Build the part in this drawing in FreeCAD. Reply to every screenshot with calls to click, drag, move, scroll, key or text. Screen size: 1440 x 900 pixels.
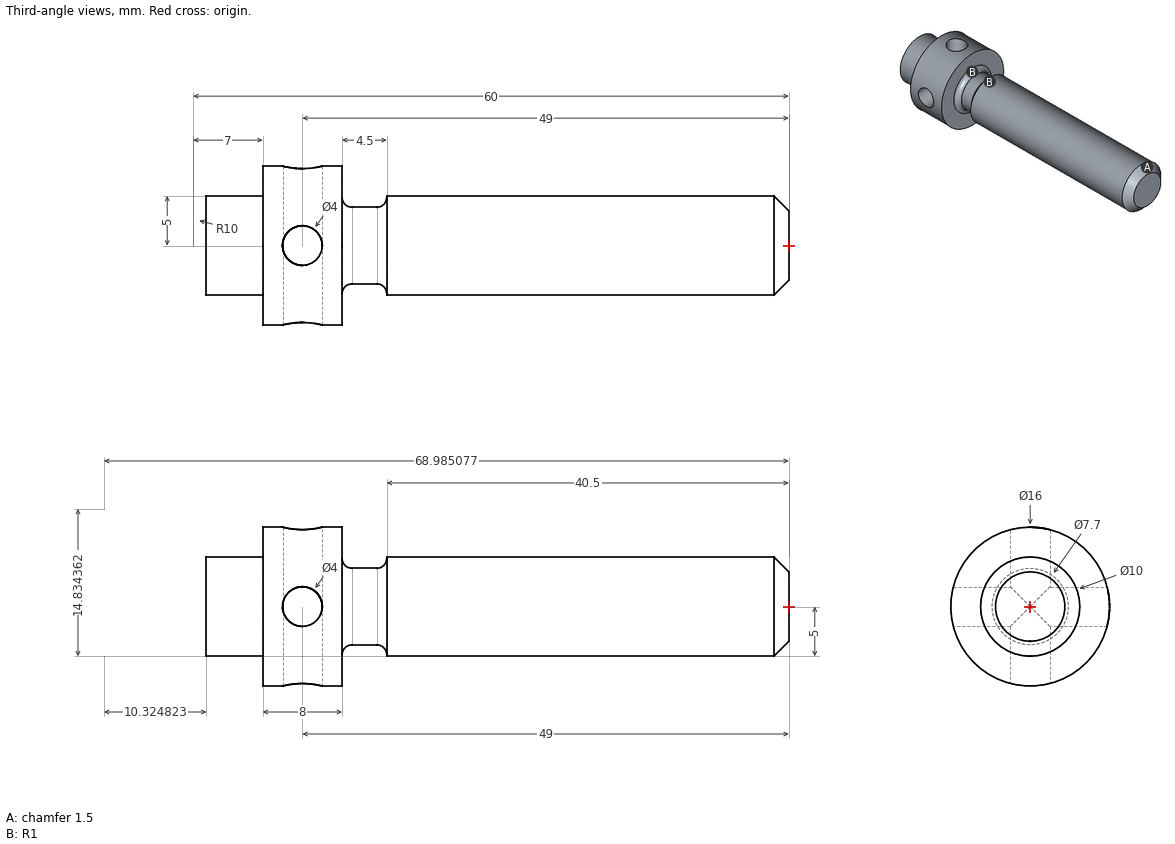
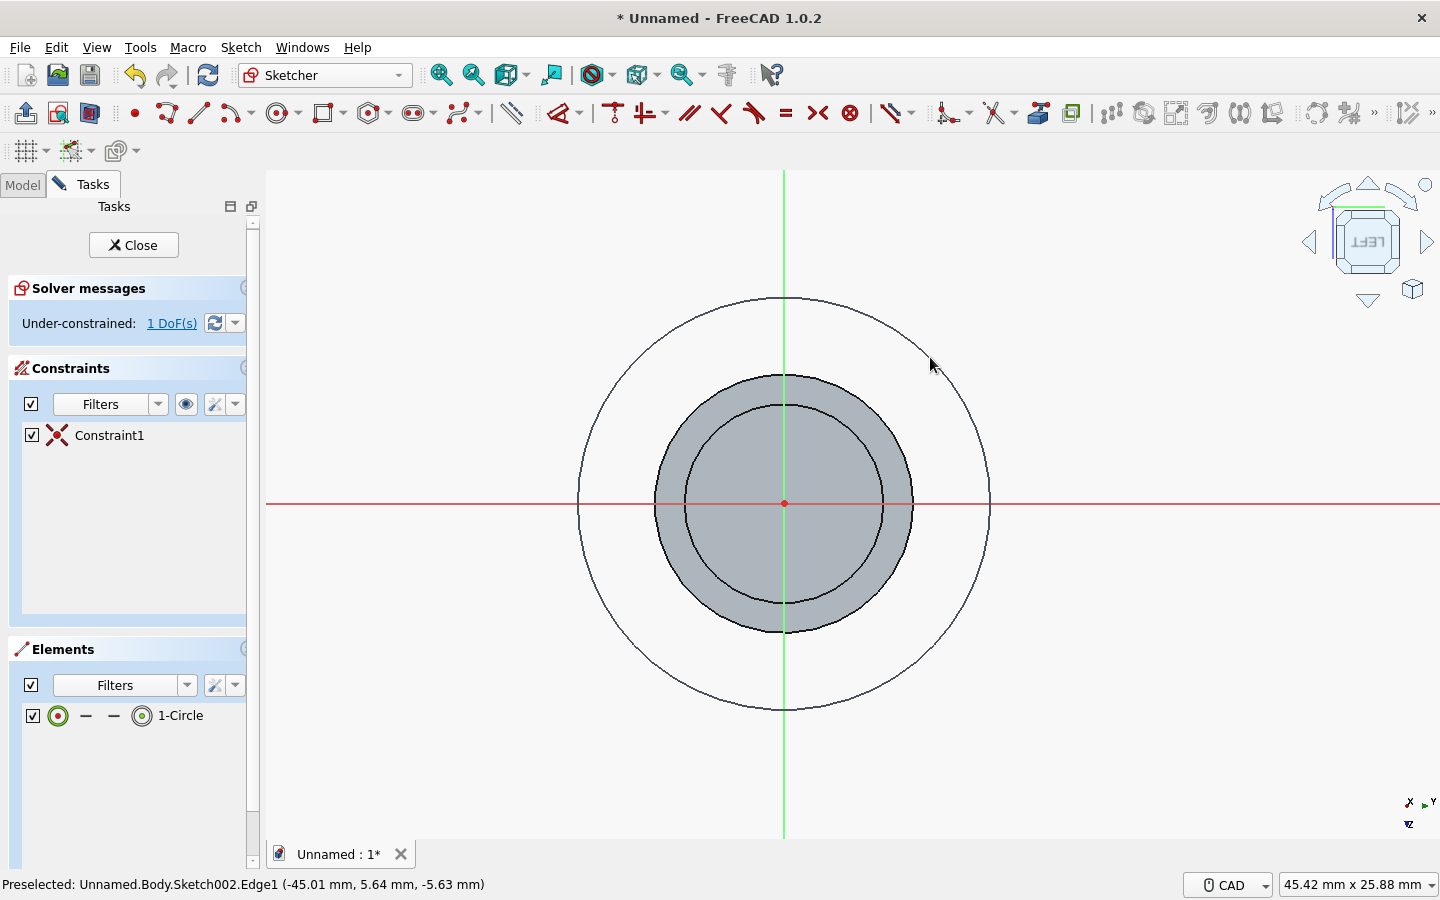
click(558, 114)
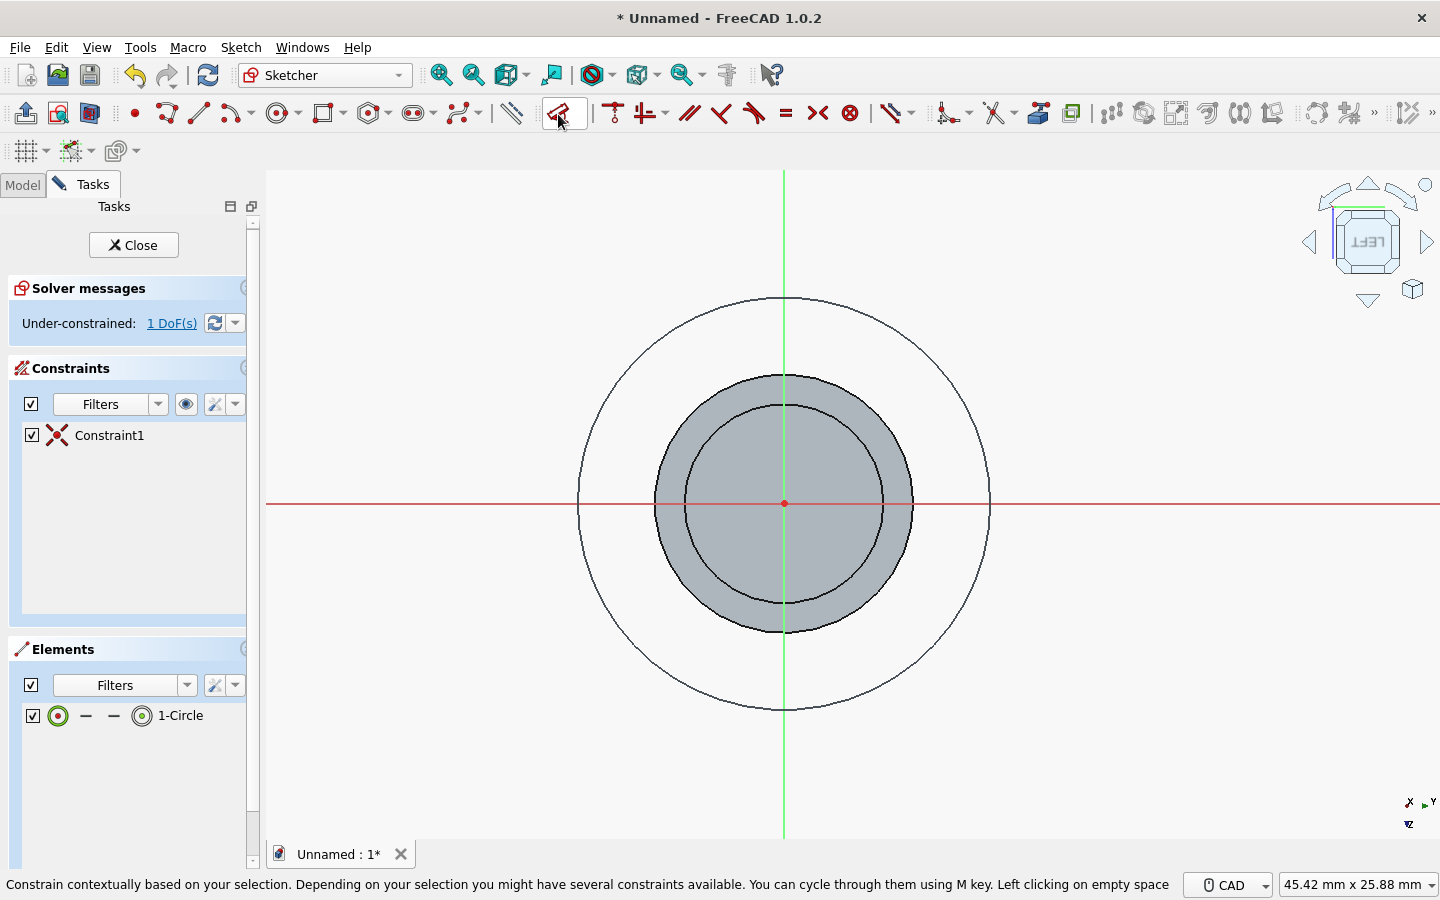
click(929, 357)
click(951, 334)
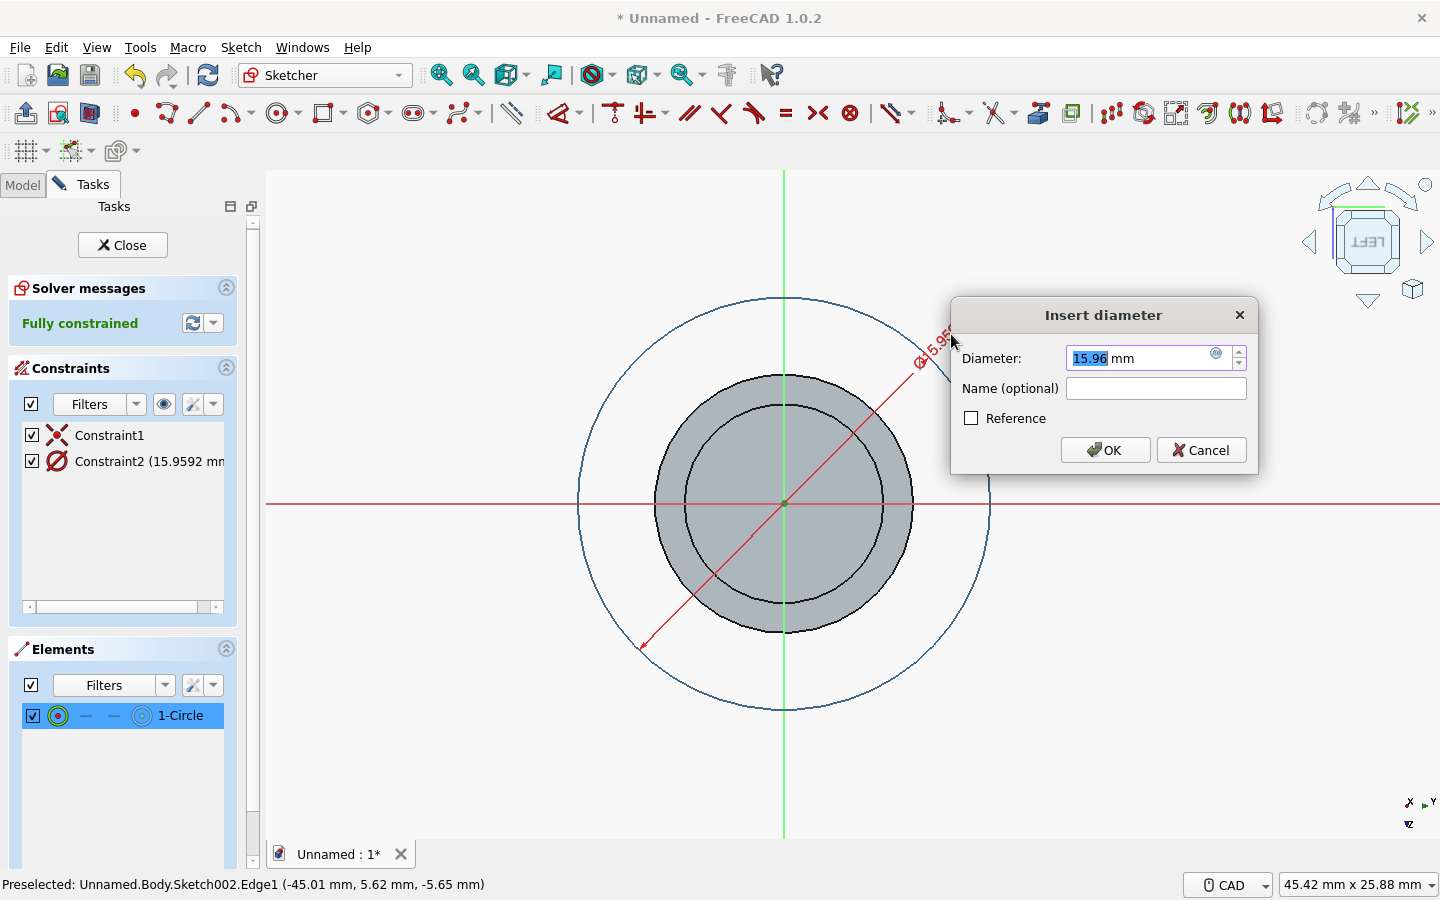
text(16)
key(Return)
key(Escape)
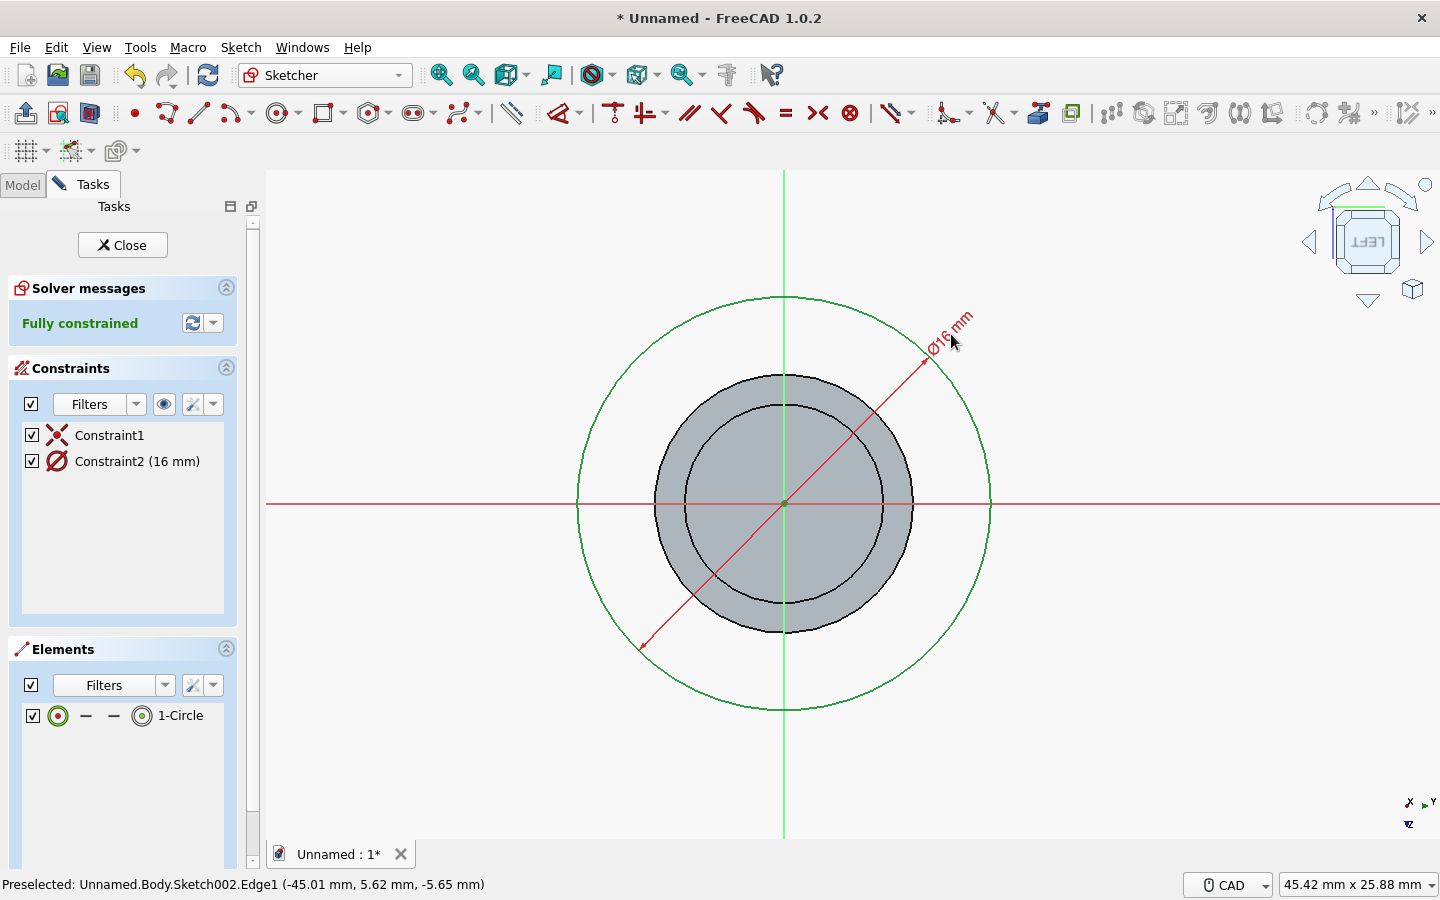
click(123, 245)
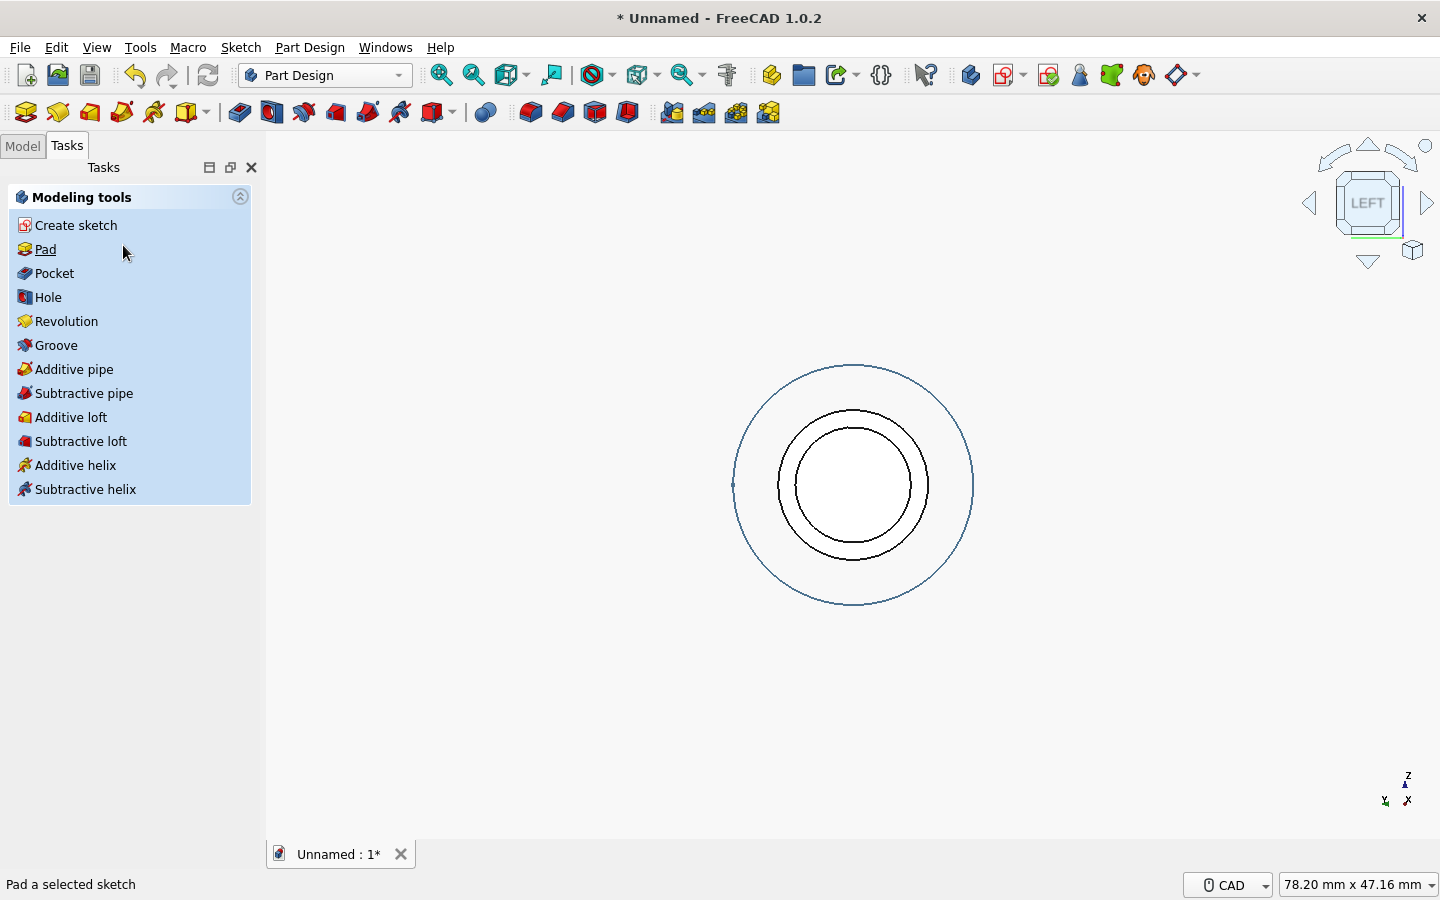
click(26, 112)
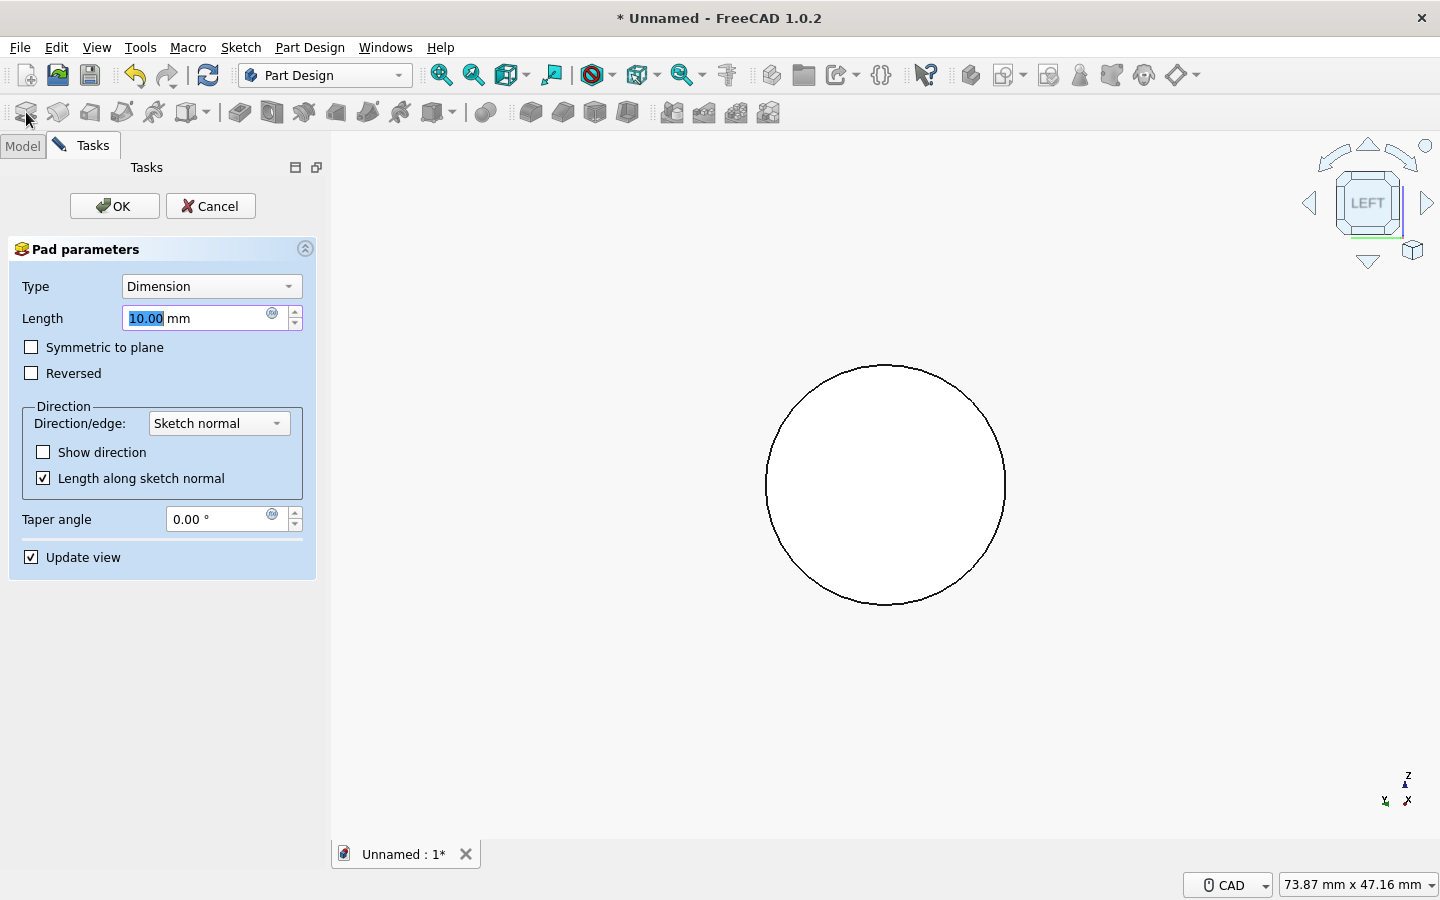
text(8)
key(Tab)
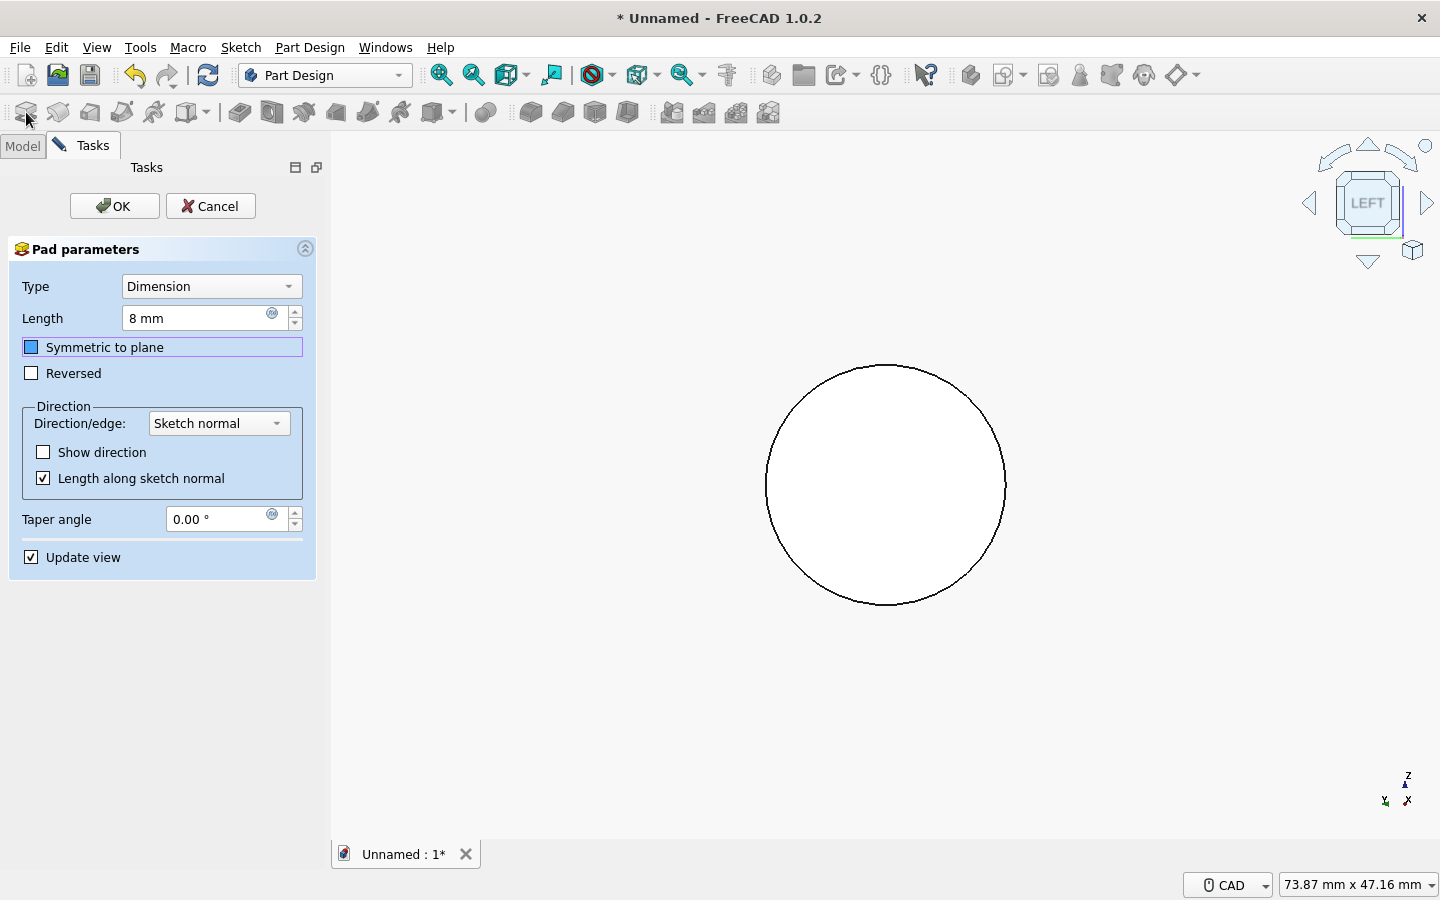
click(115, 206)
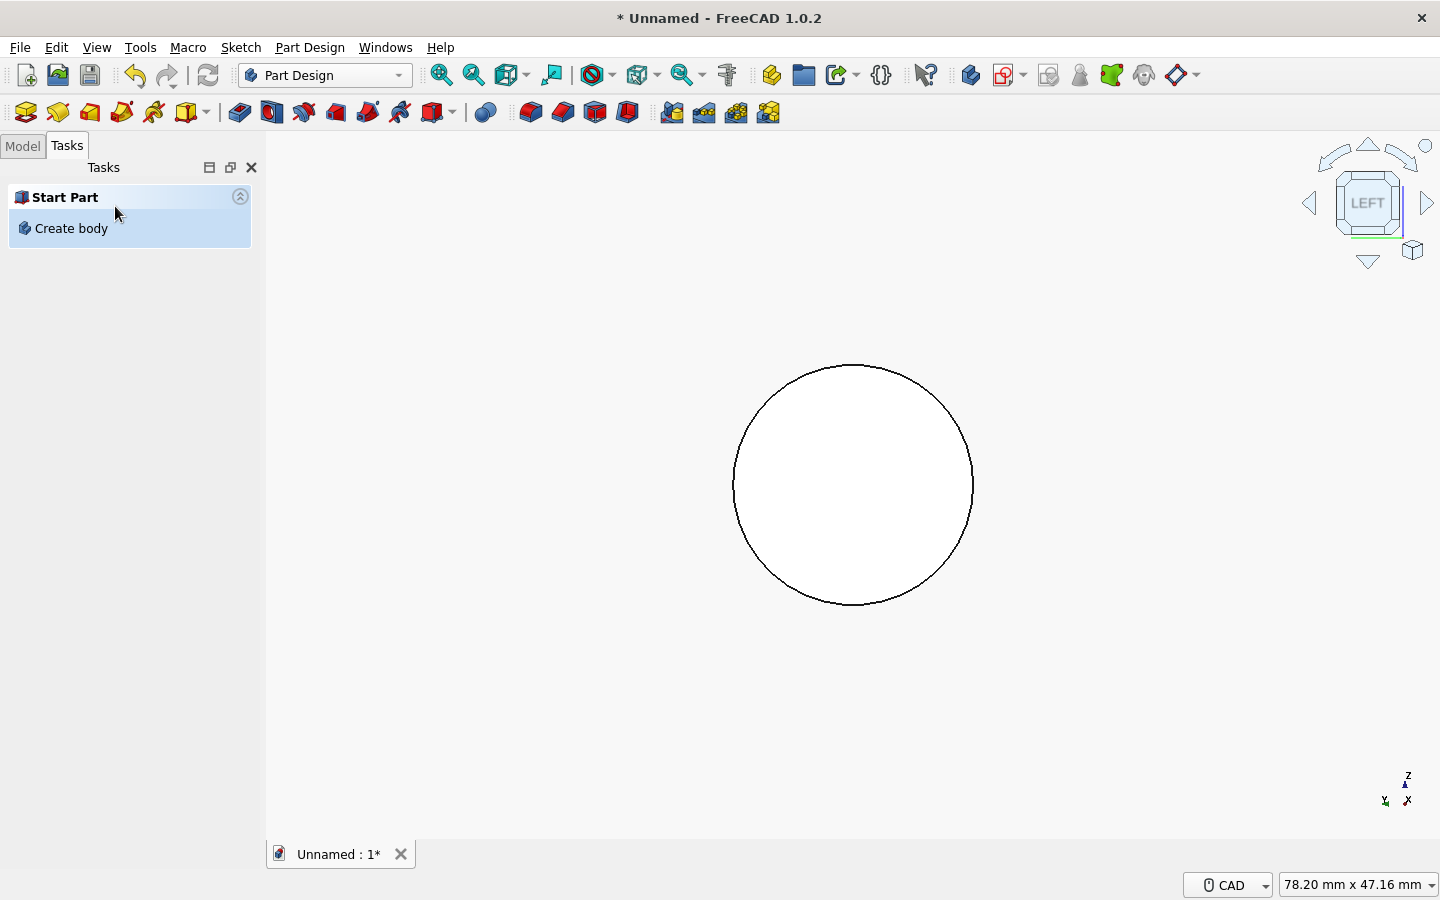
key(v)
key(f)